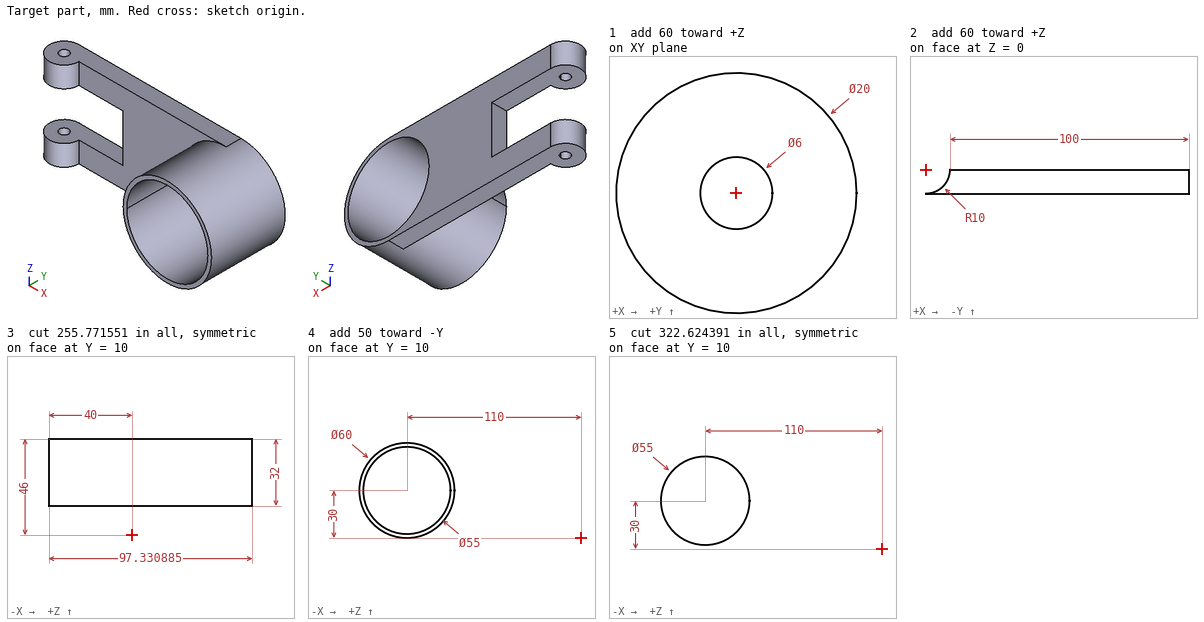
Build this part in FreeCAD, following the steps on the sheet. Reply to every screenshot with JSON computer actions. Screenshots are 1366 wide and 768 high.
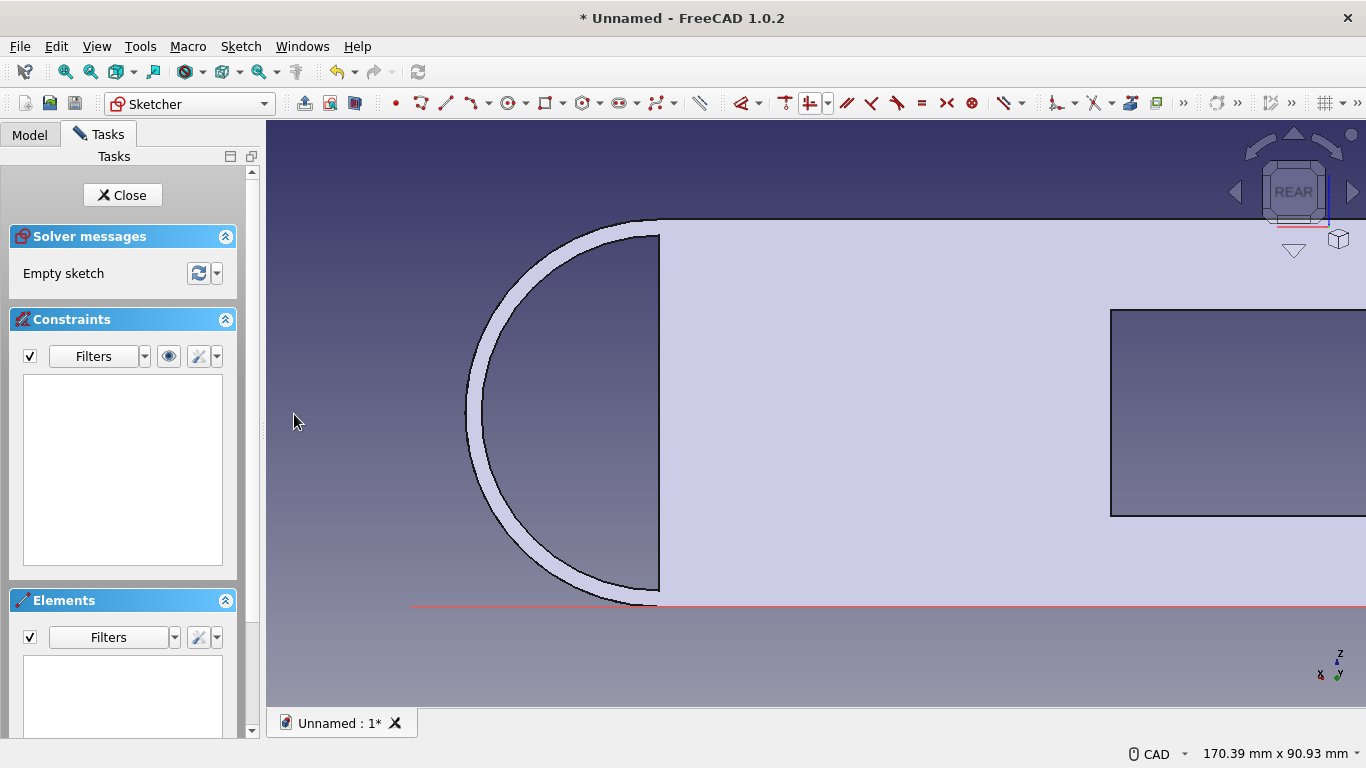
{"action": "left_click", "coordinate": [508, 104]}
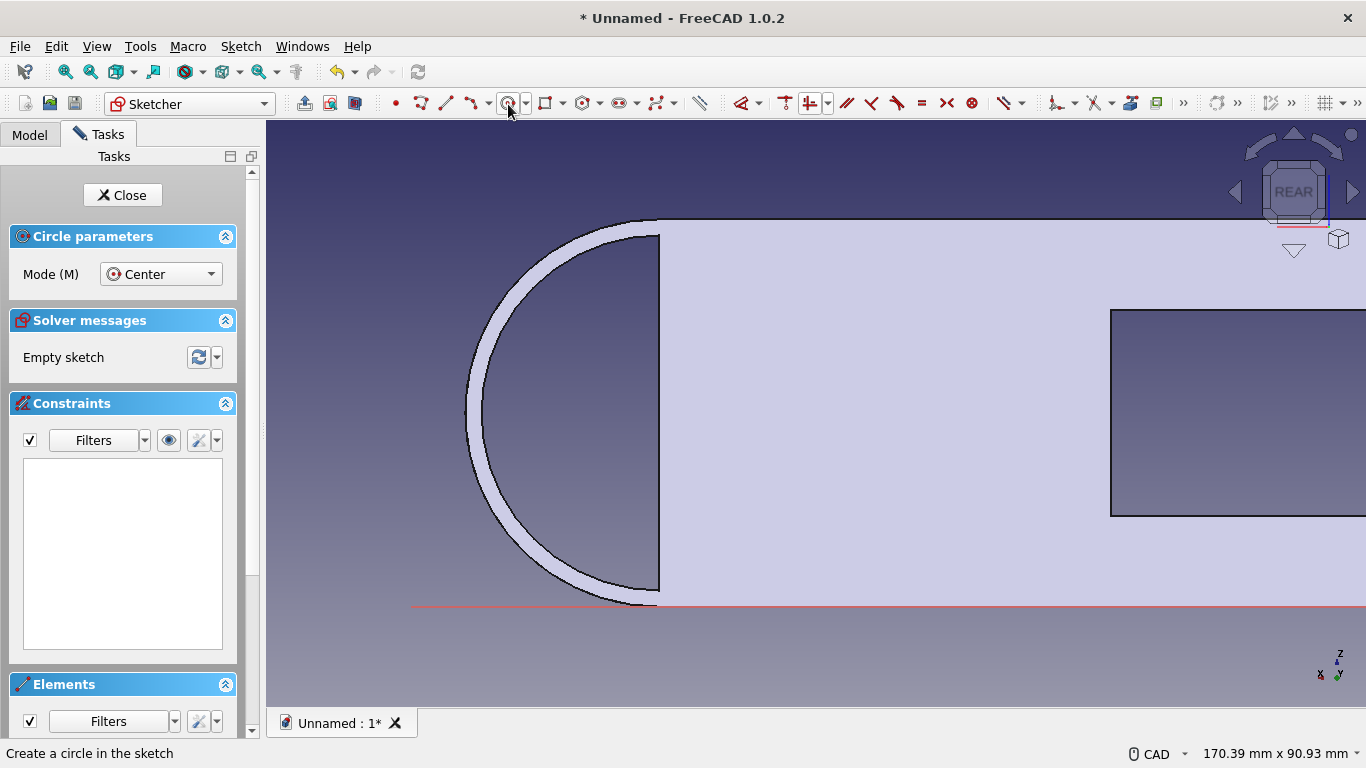
{"action": "left_click", "coordinate": [659, 413]}
{"action": "mouse_move", "coordinate": [785, 287]}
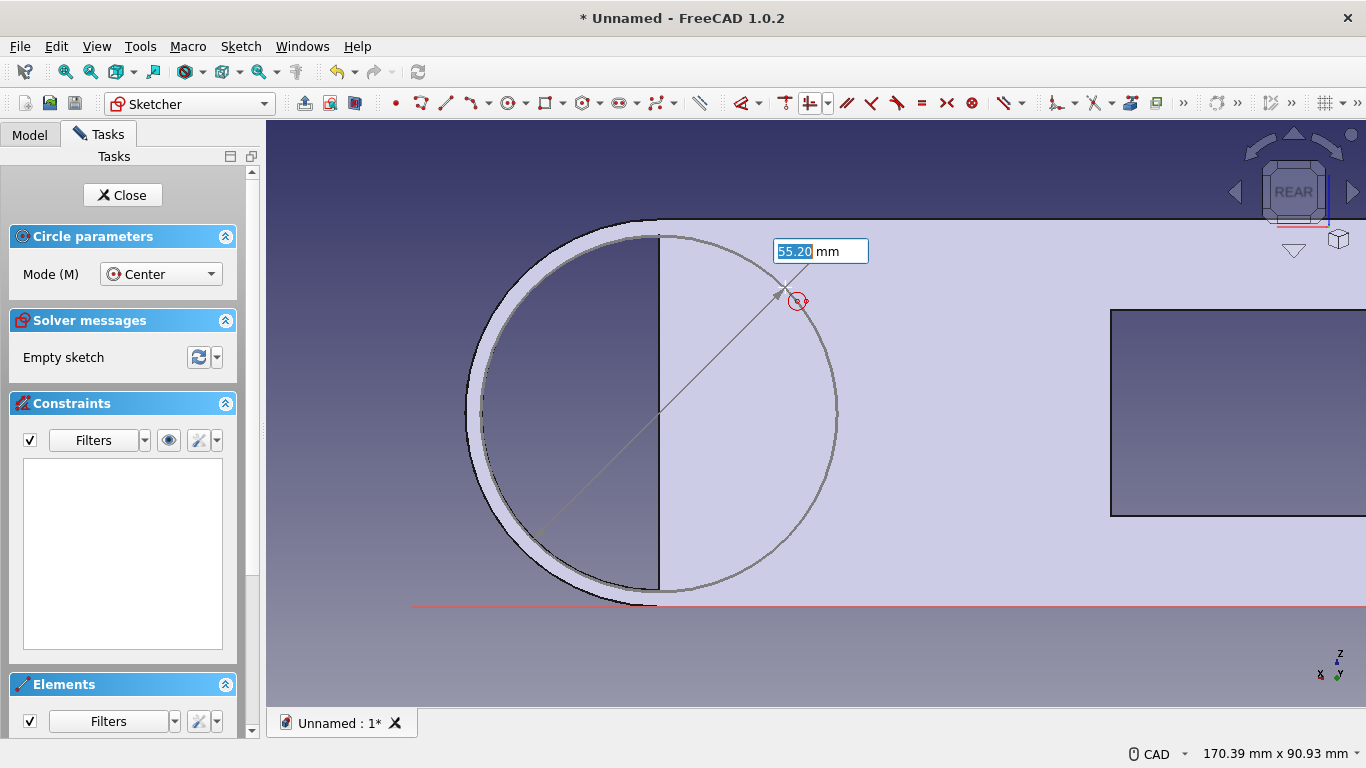
{"action": "type", "text": "55"}
{"action": "key", "text": "Return"}
{"action": "key", "text": "Escape"}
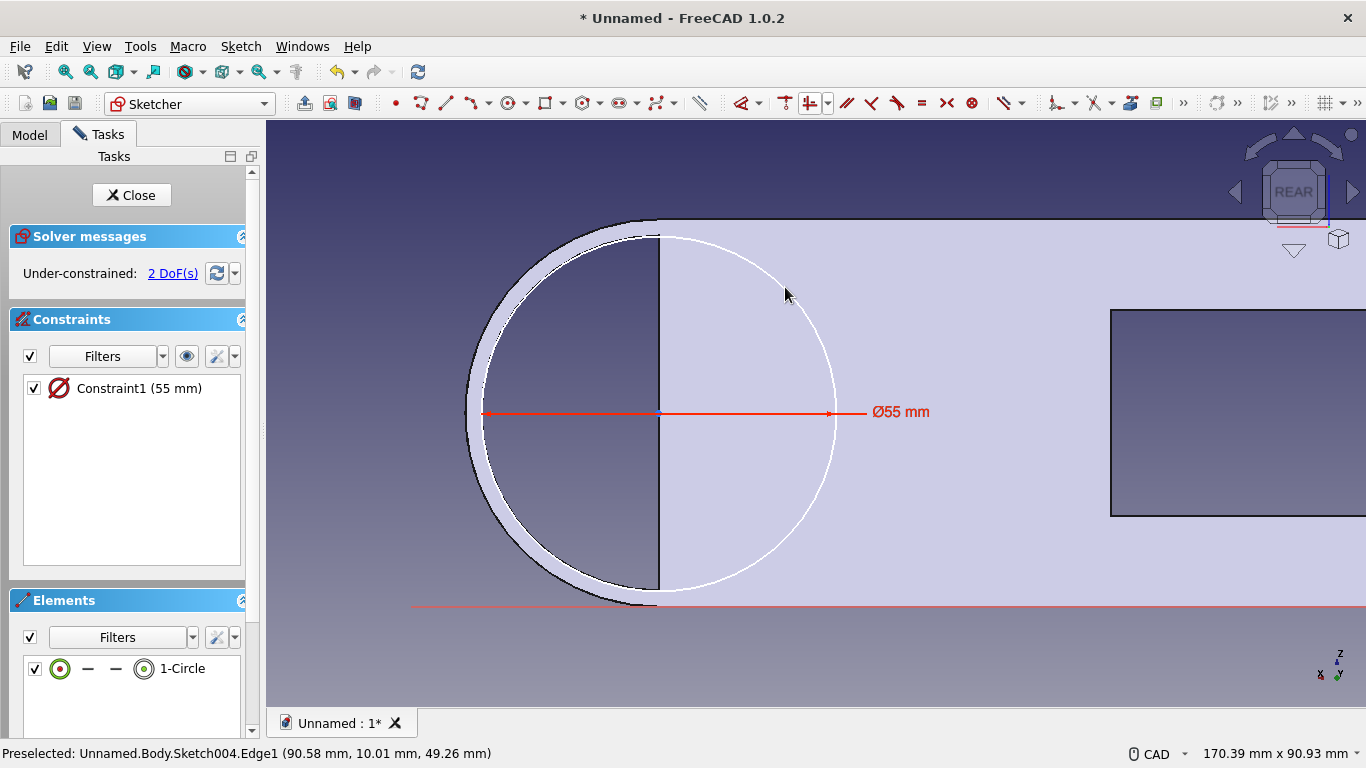
{"action": "left_click", "coordinate": [740, 104]}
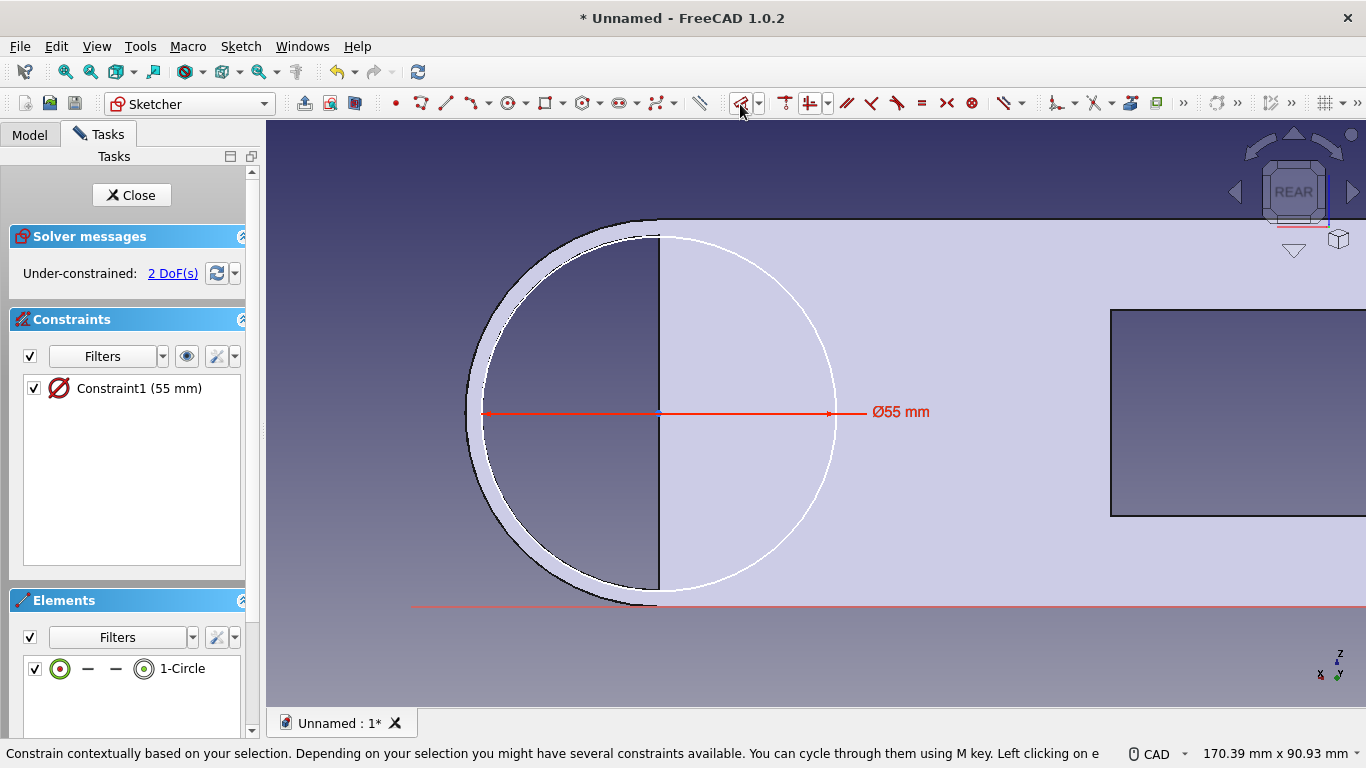
{"action": "left_click", "coordinate": [659, 414]}
{"action": "left_click", "coordinate": [625, 510]}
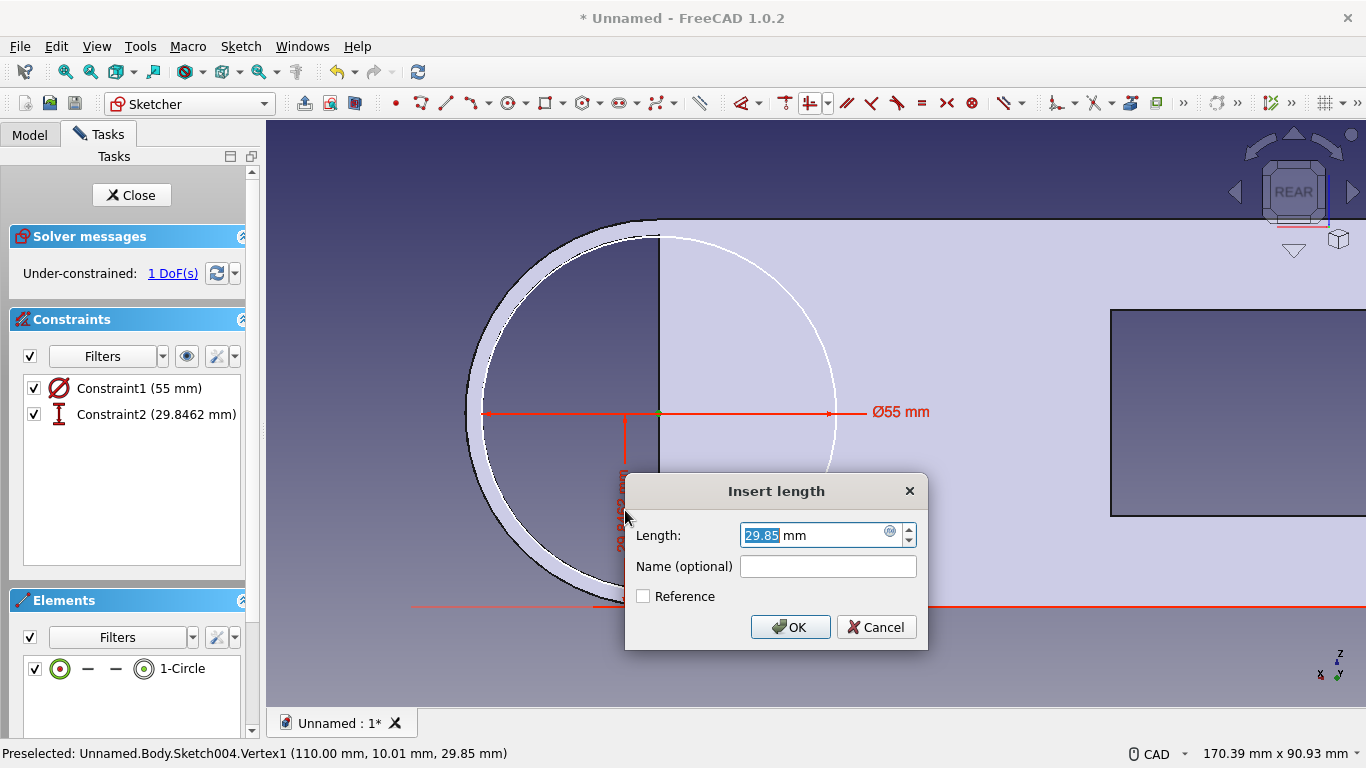
{"action": "type", "text": "30"}
{"action": "key", "text": "Return"}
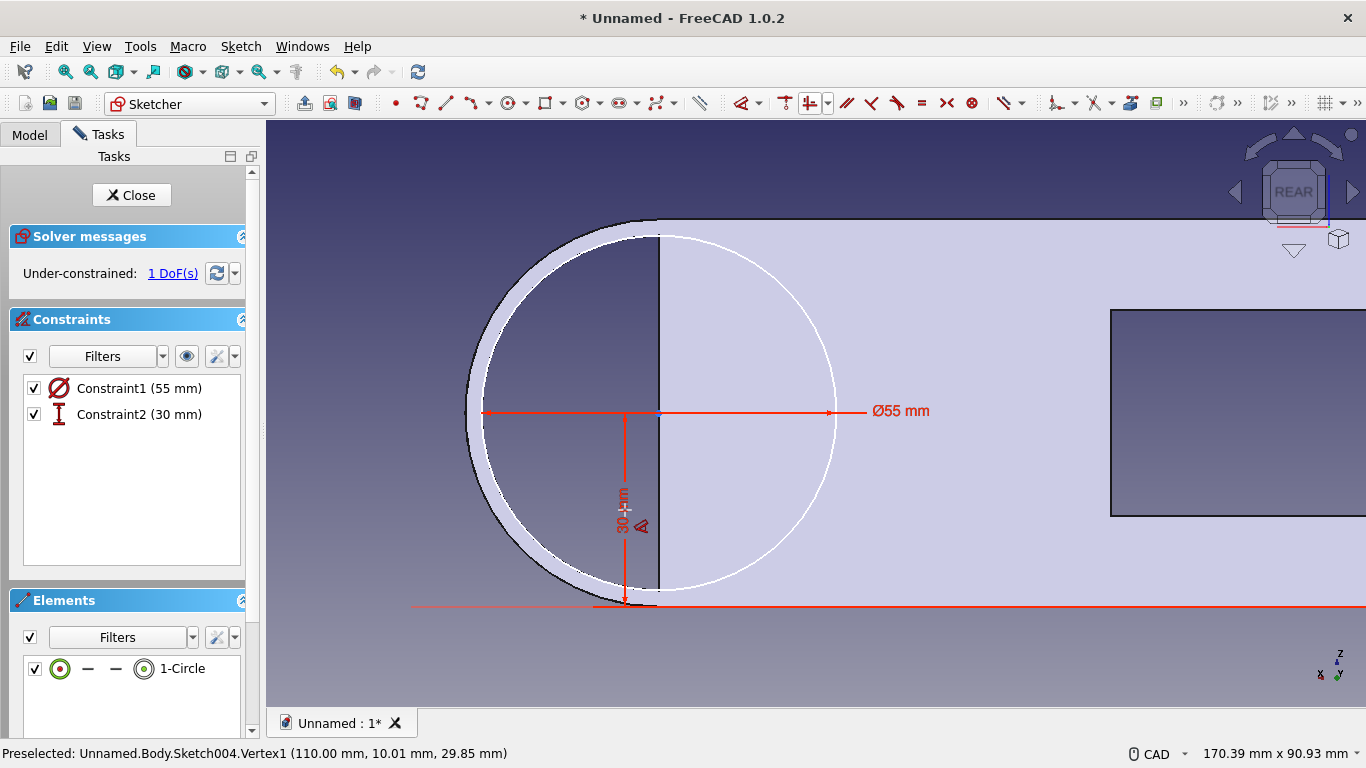
{"action": "left_click", "coordinate": [659, 413]}
{"action": "left_click", "coordinate": [930, 641]}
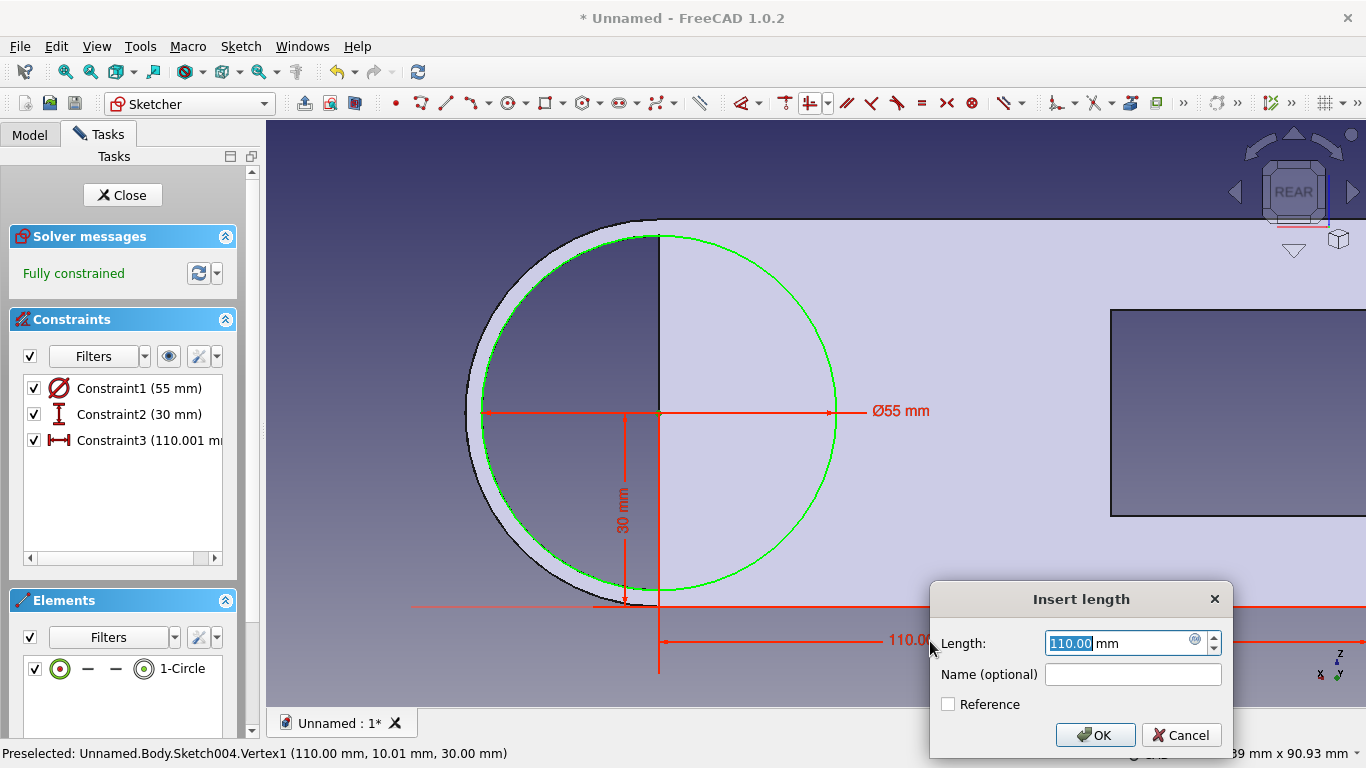
{"action": "type", "text": "110"}
{"action": "key", "text": "Return"}
{"action": "key", "text": "Escape"}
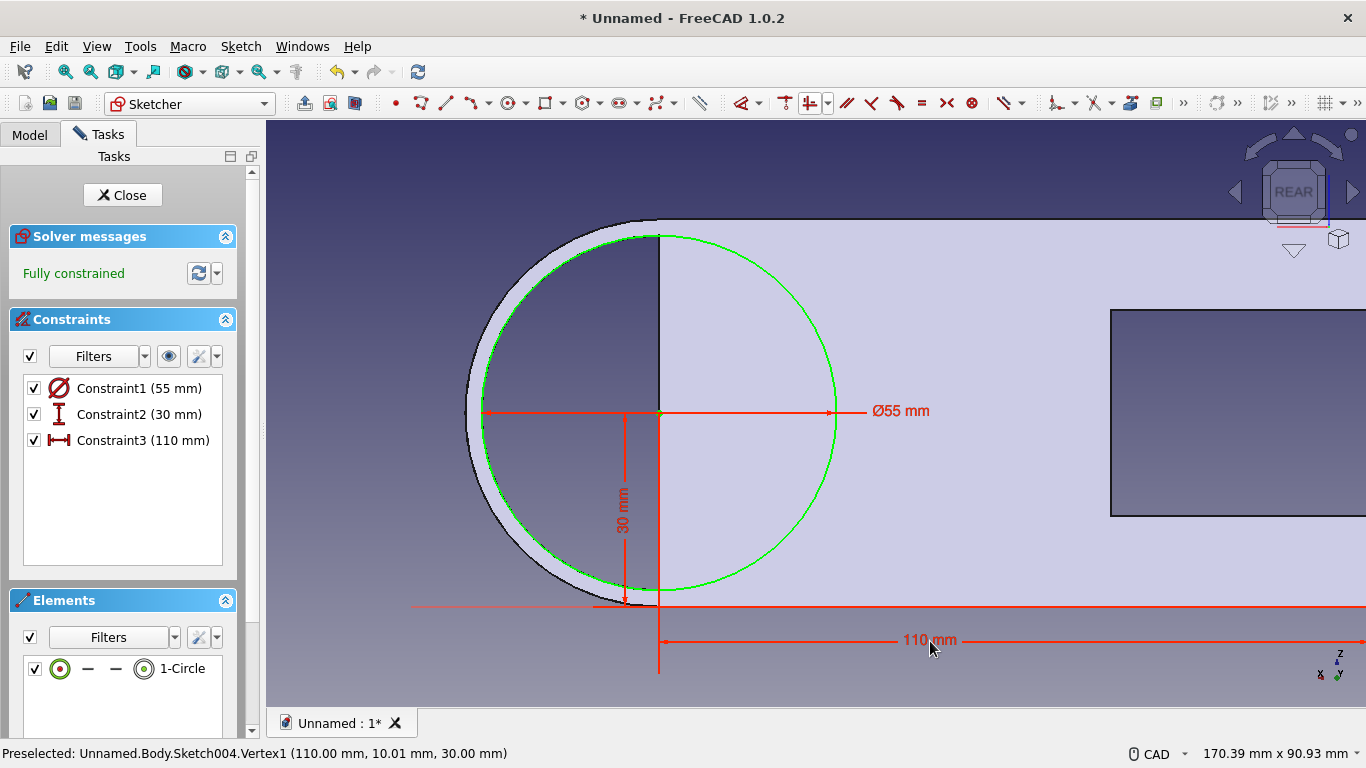
{"action": "left_click", "coordinate": [123, 195]}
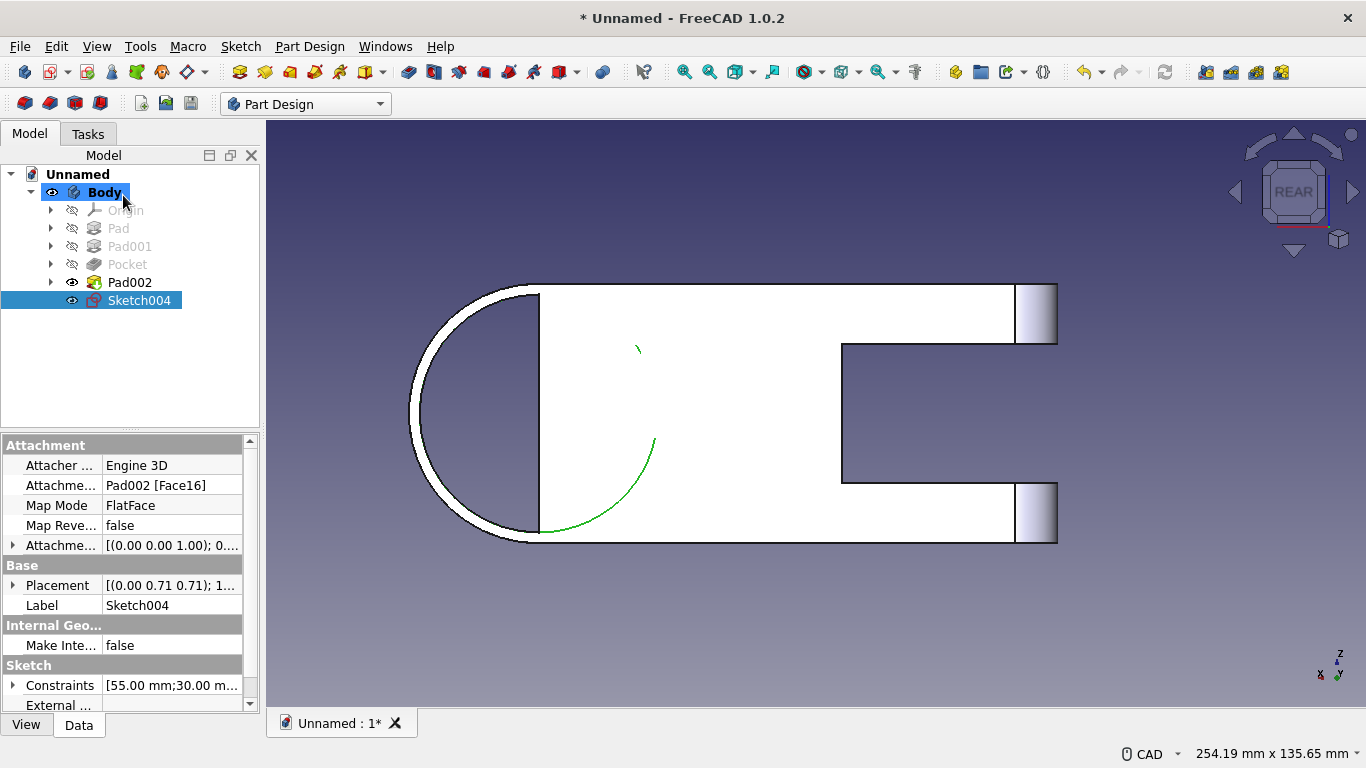
{"action": "left_click", "coordinate": [409, 72]}